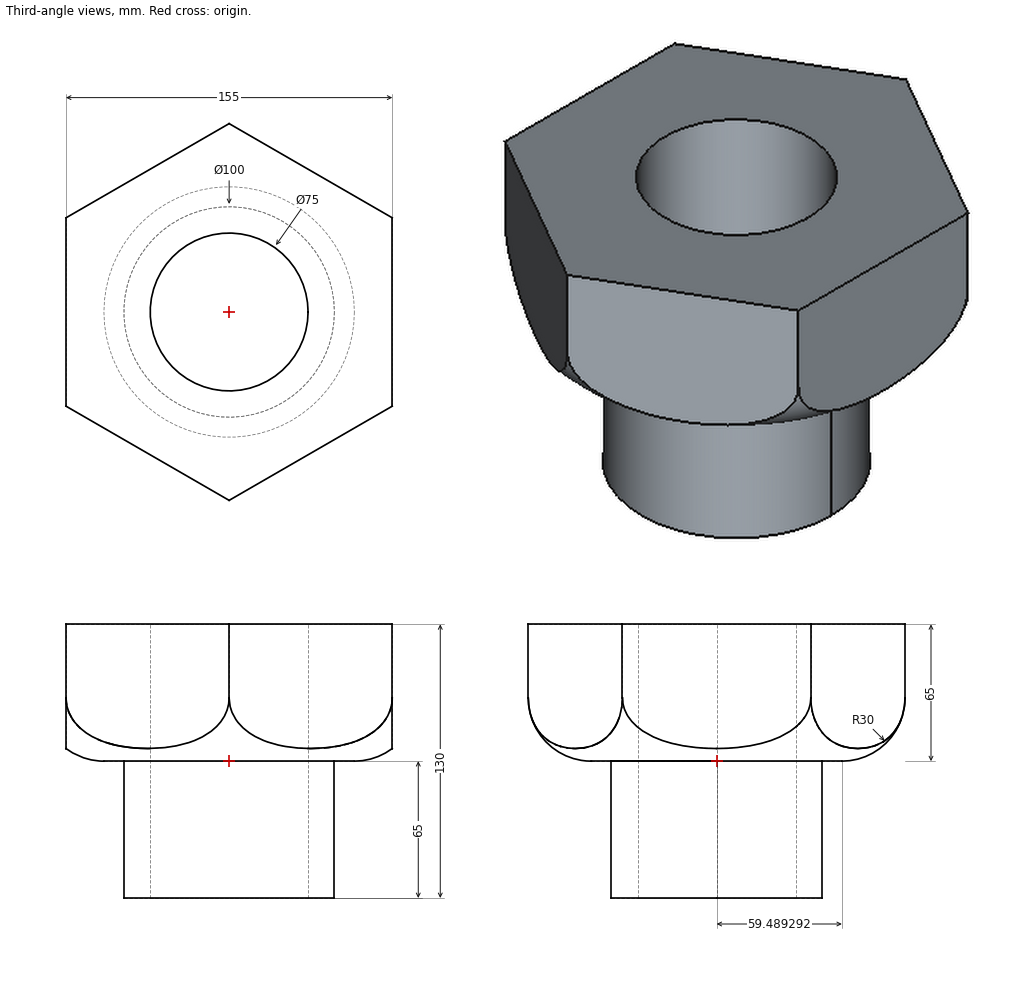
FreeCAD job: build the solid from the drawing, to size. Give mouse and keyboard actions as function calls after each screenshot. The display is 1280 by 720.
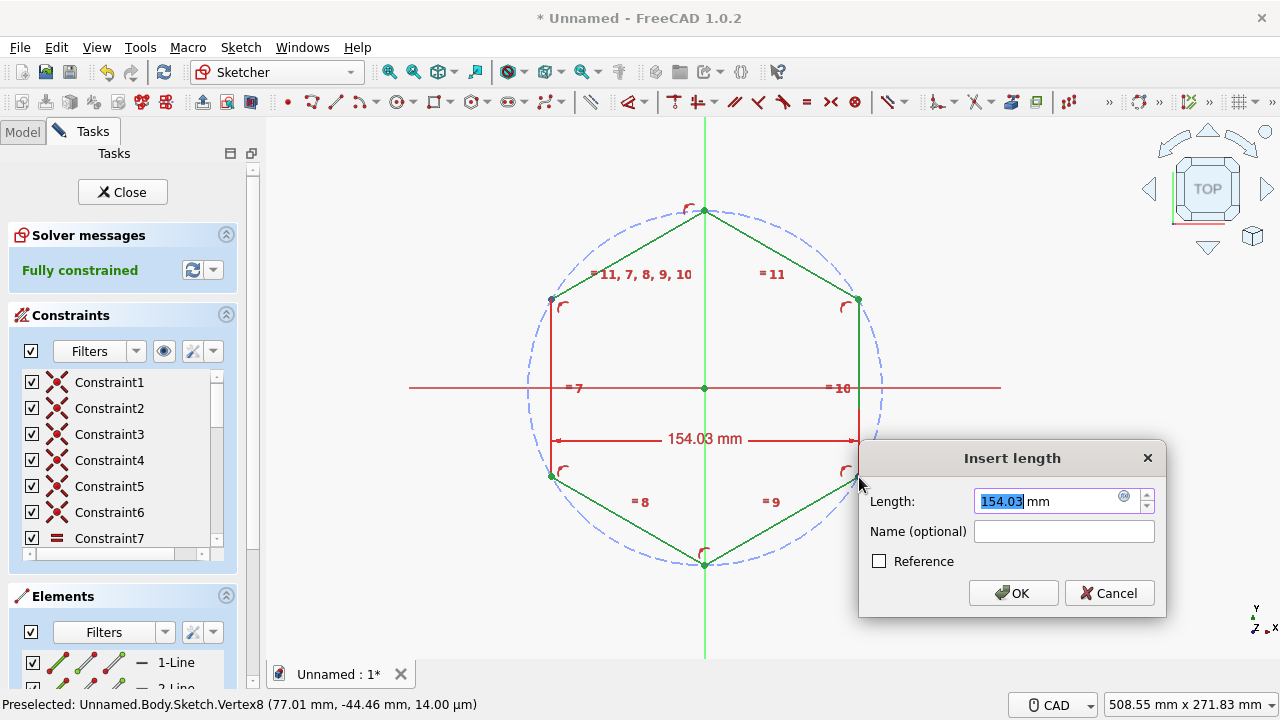
text(155)
key(Return)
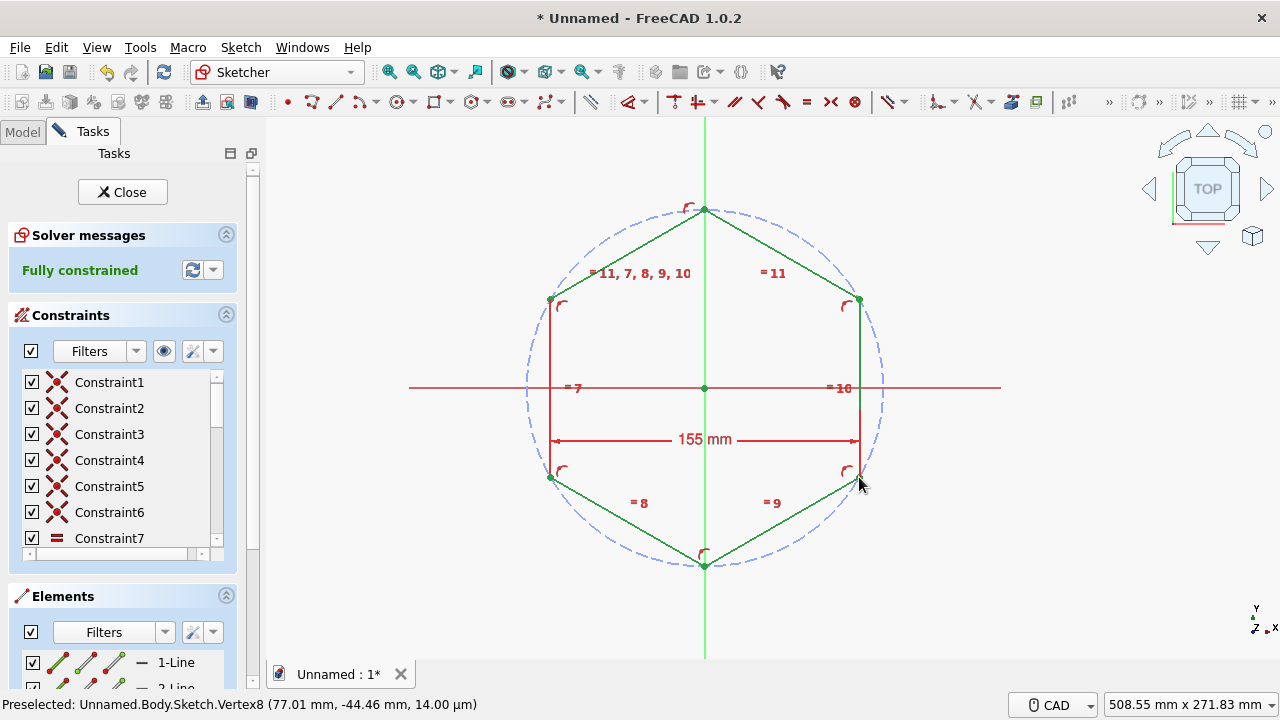
click(123, 192)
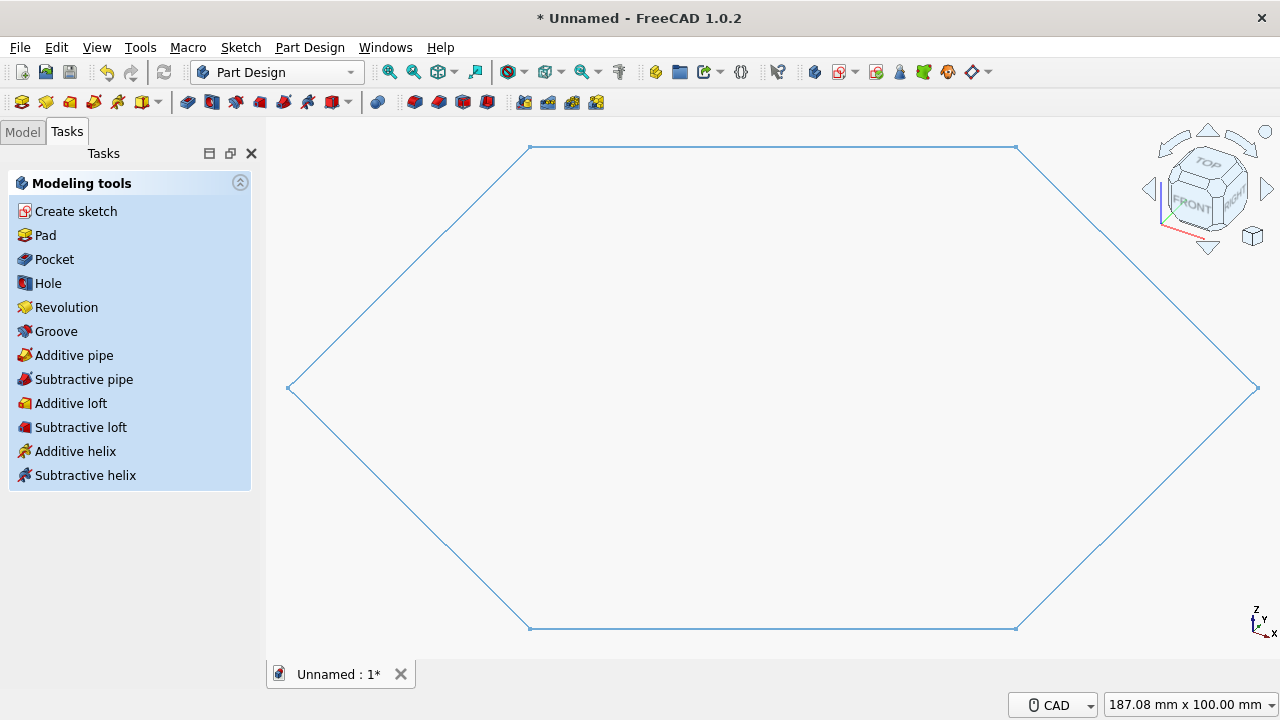
click(22, 102)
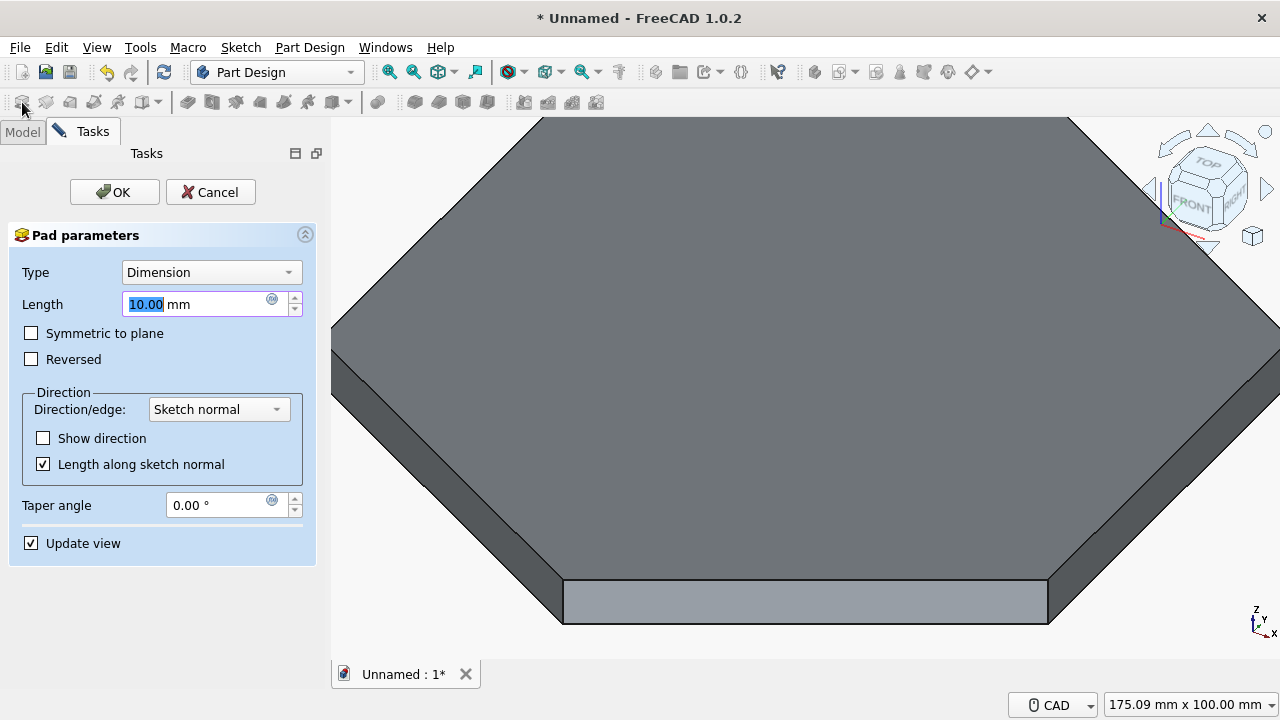
text(65)
key(Tab)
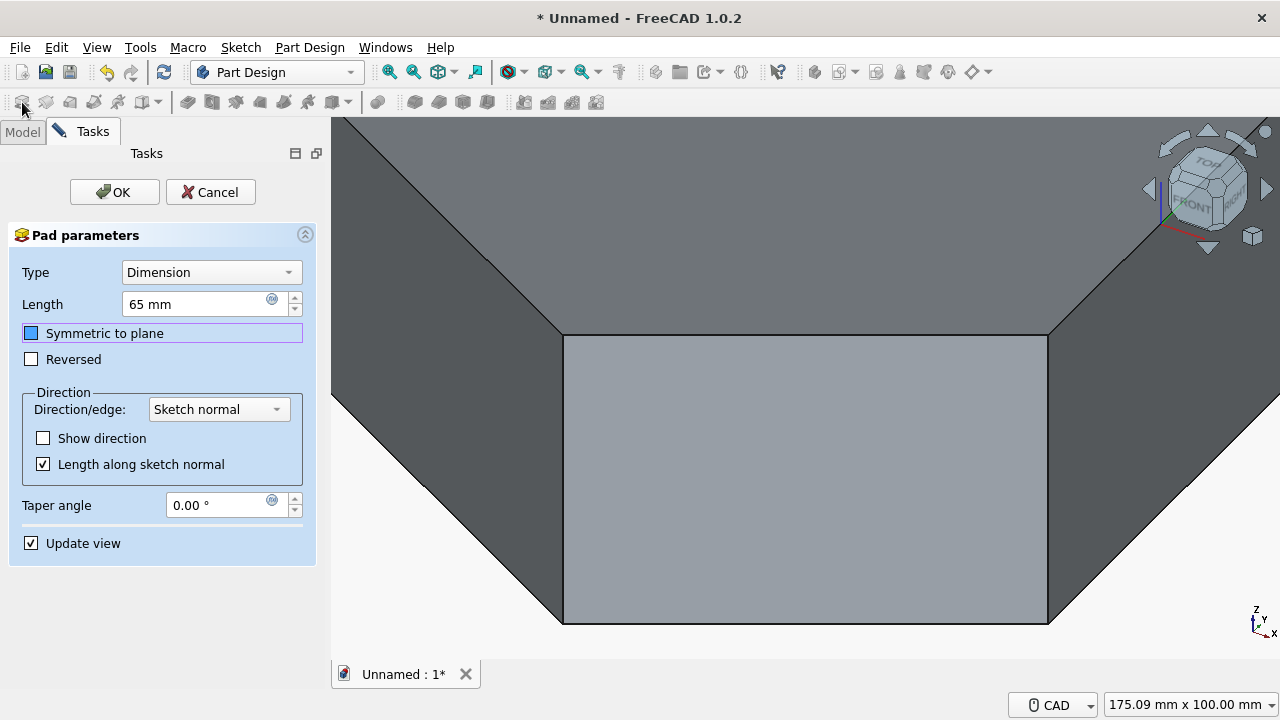
click(115, 192)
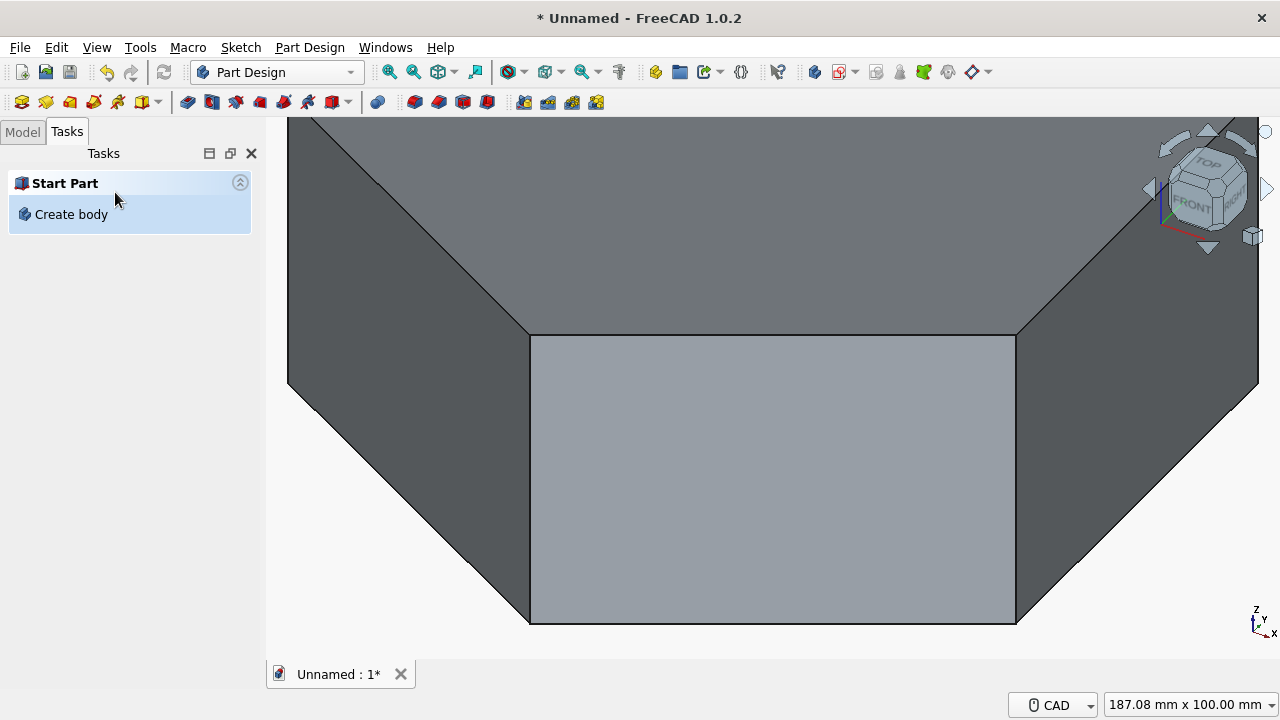
key(v)
key(f)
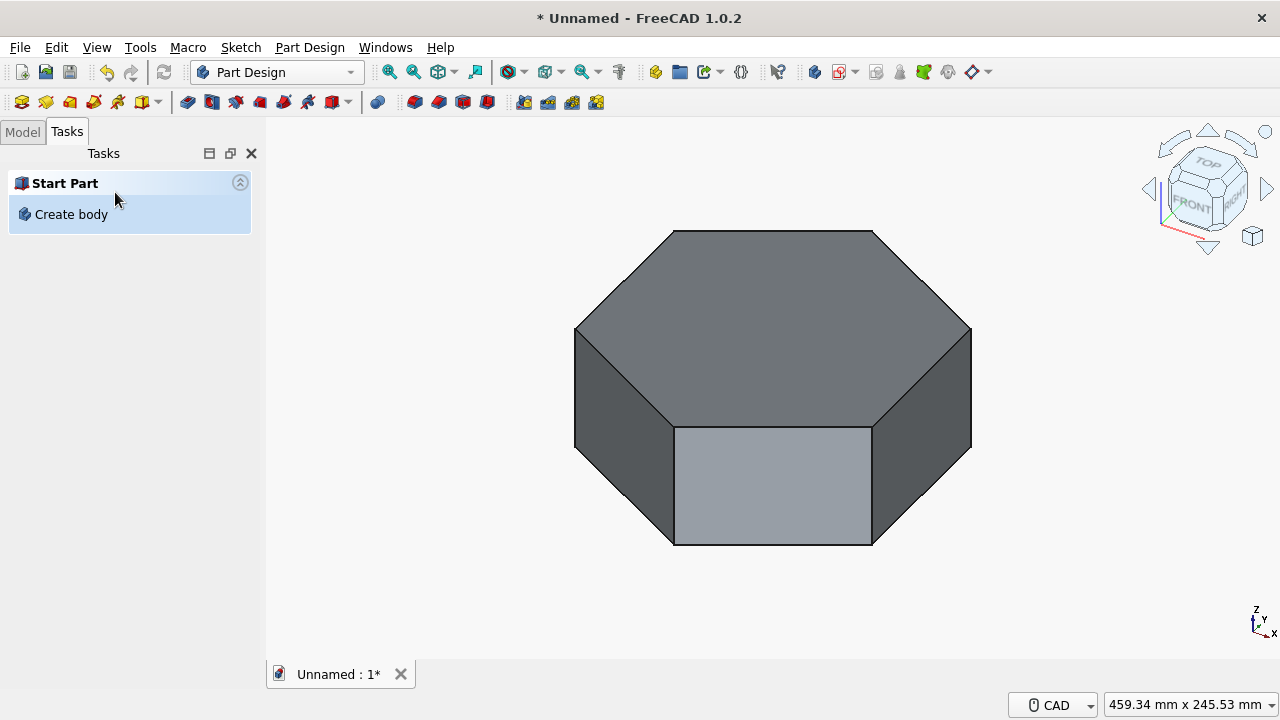
click(840, 72)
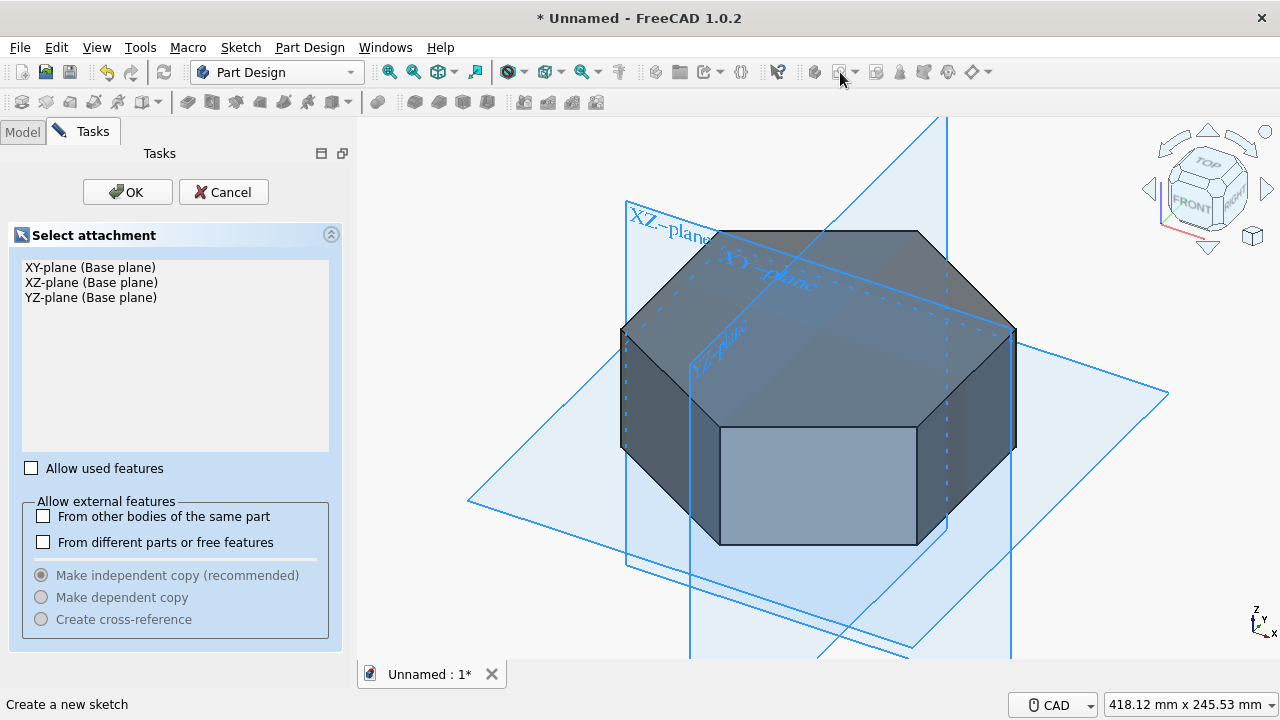
click(82, 298)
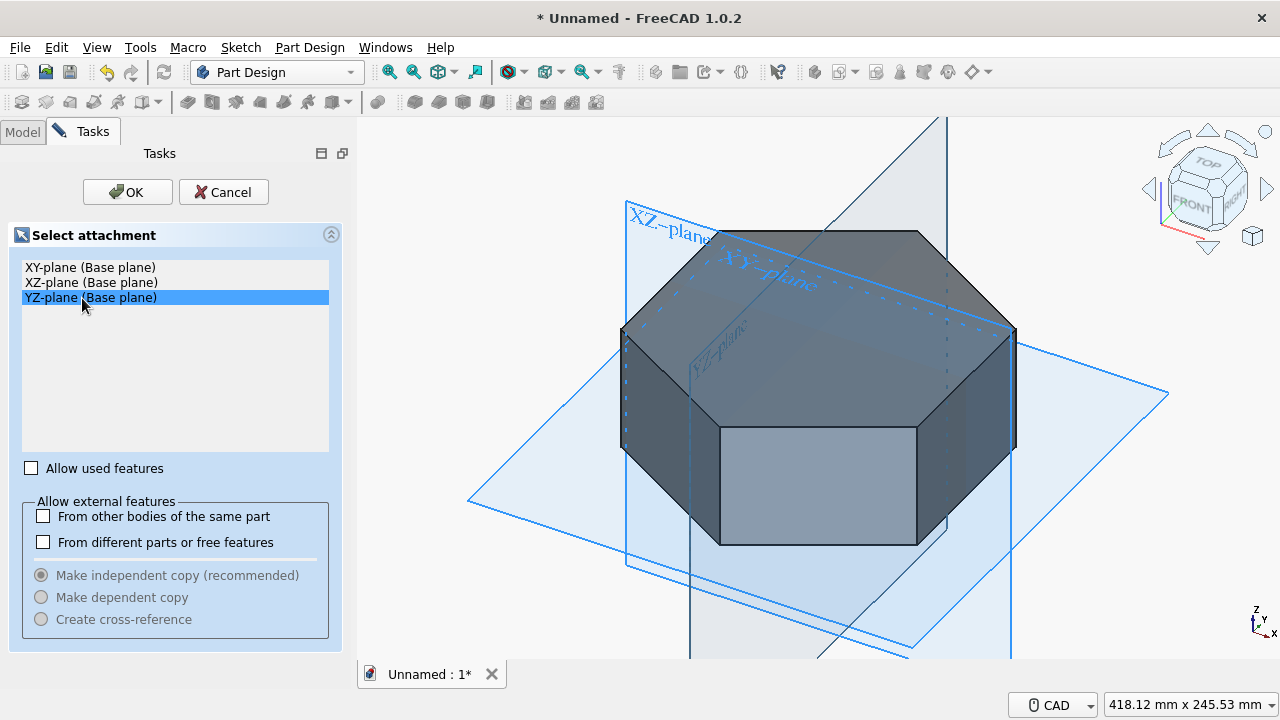
click(128, 192)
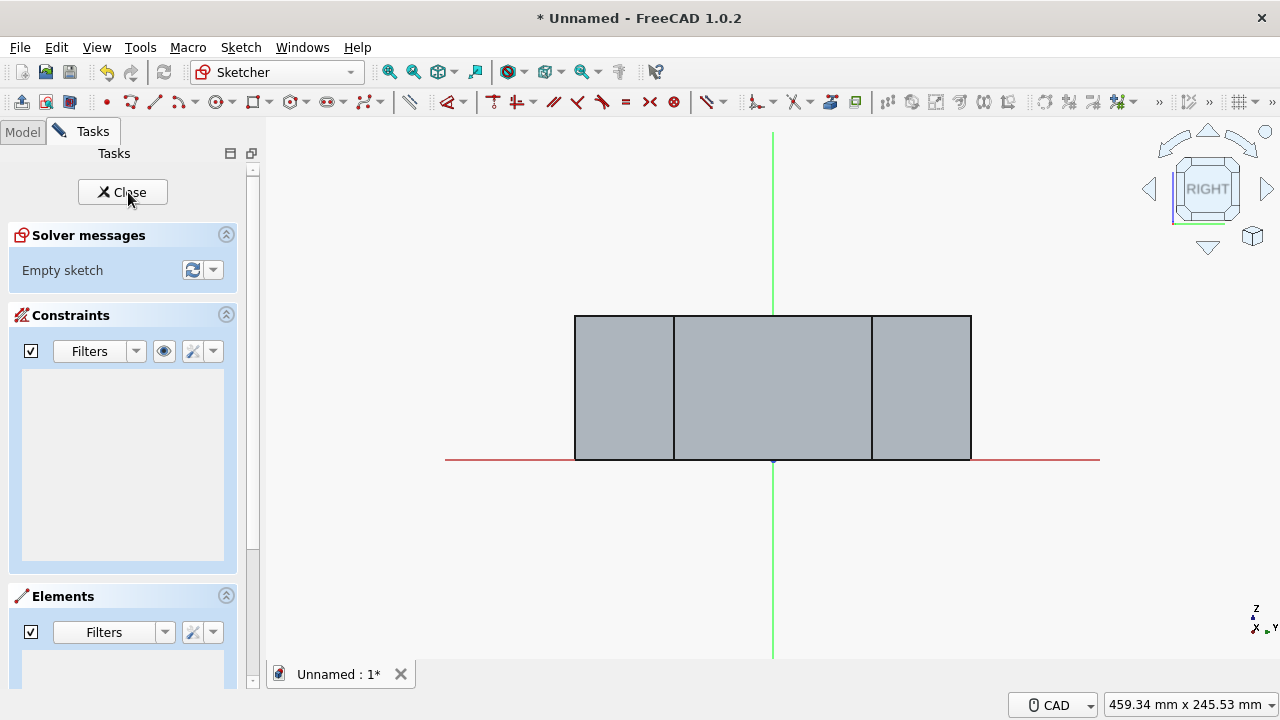
click(70, 102)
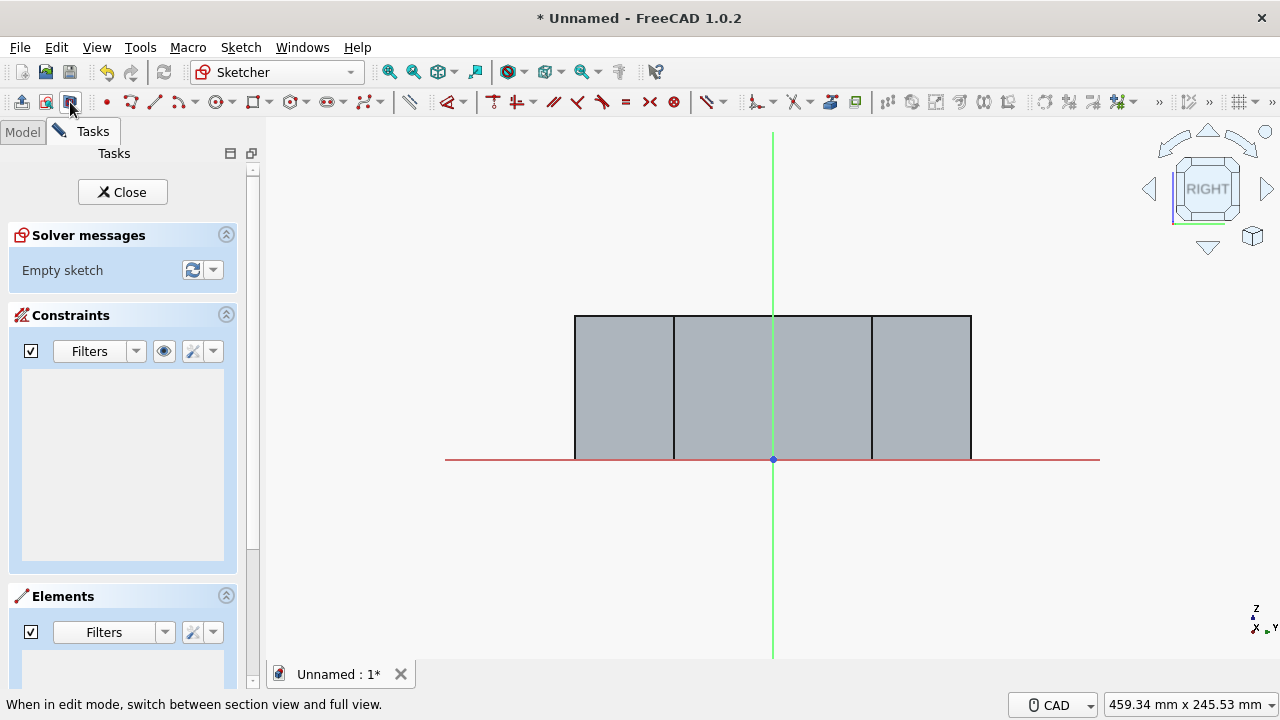
scroll(996, 436, up, 8)